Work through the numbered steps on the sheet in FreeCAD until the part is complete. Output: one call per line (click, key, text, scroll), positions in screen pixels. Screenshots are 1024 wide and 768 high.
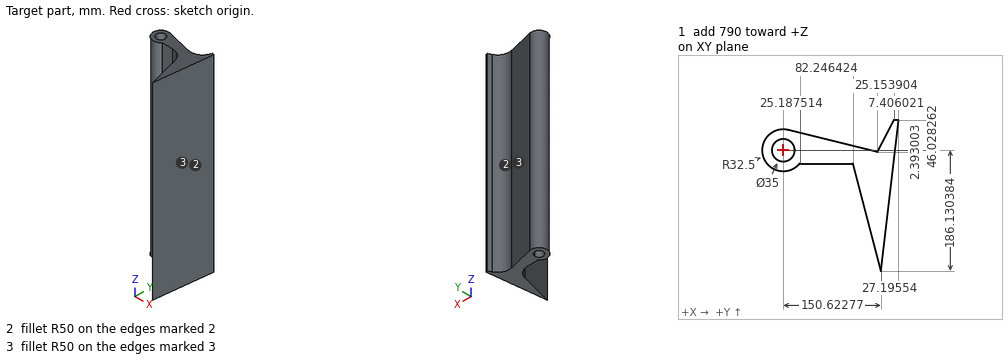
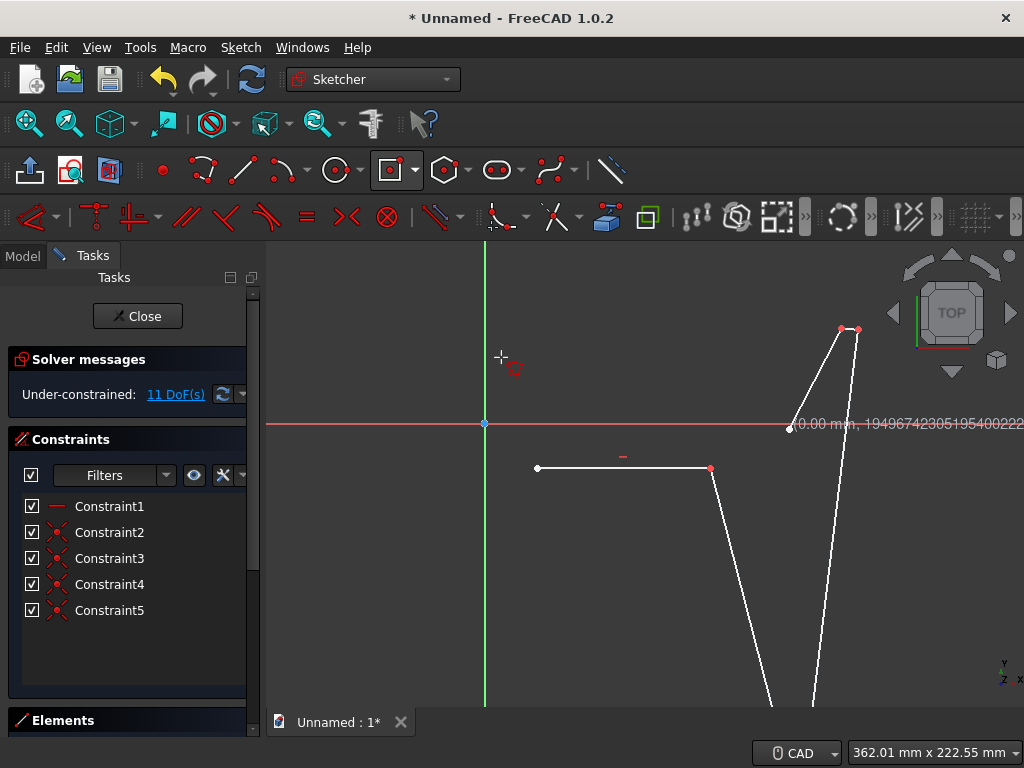
click(501, 358)
right_click(501, 358)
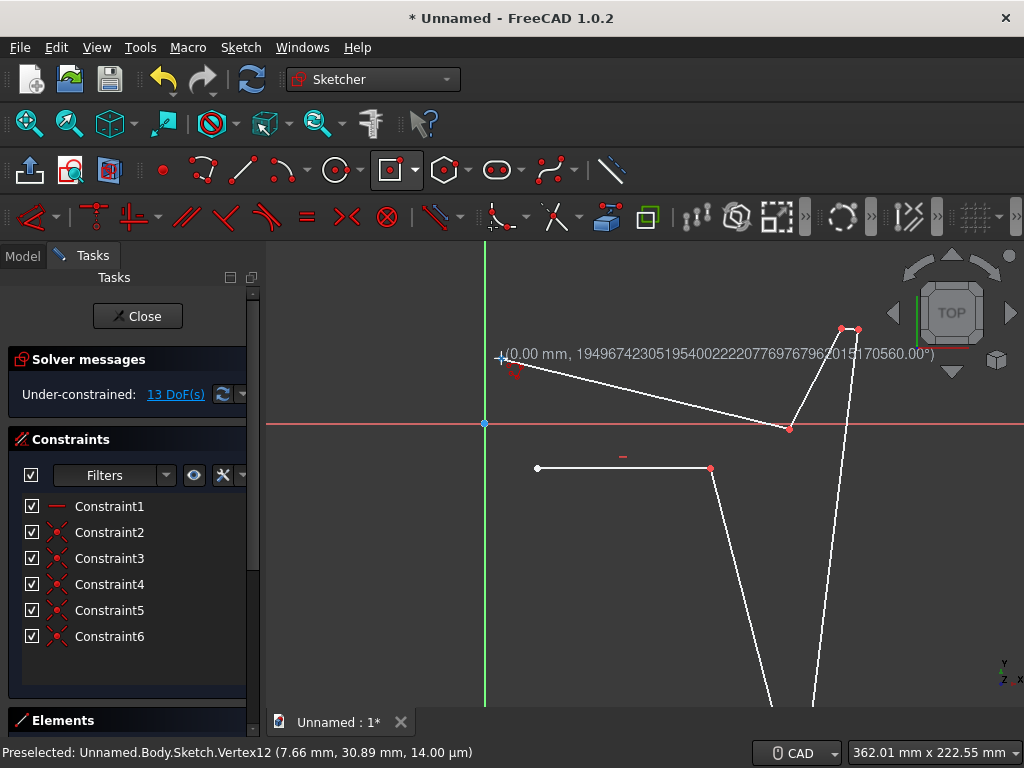
key(g)
key(3)
key(a)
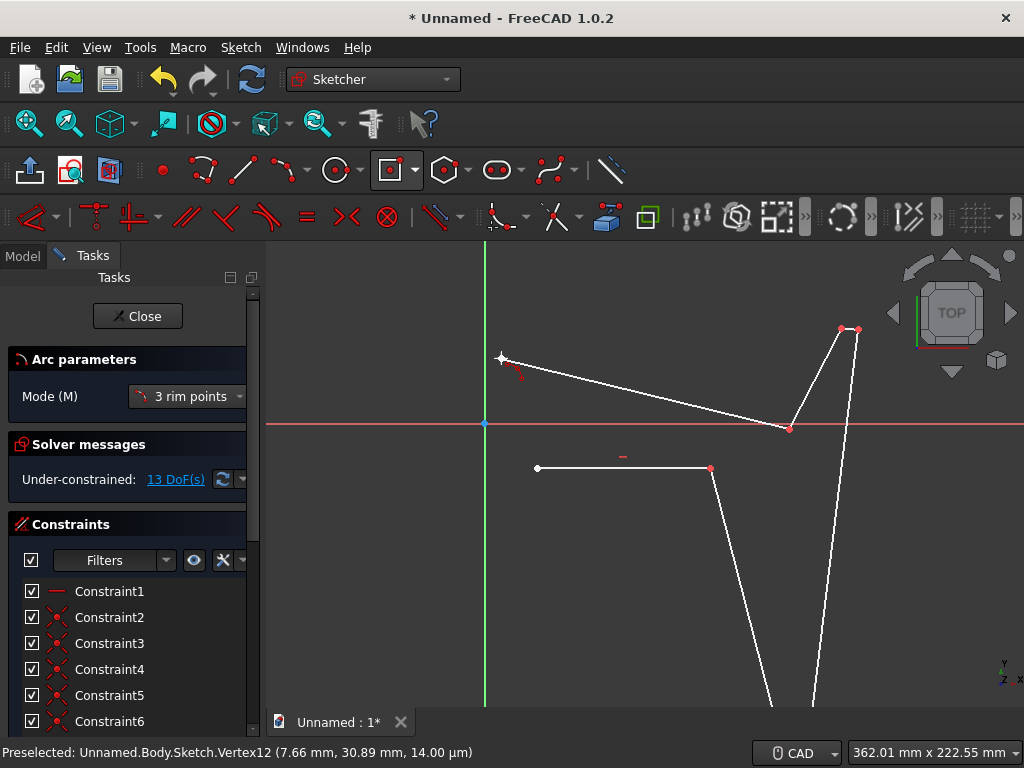
click(501, 359)
click(537, 468)
click(435, 470)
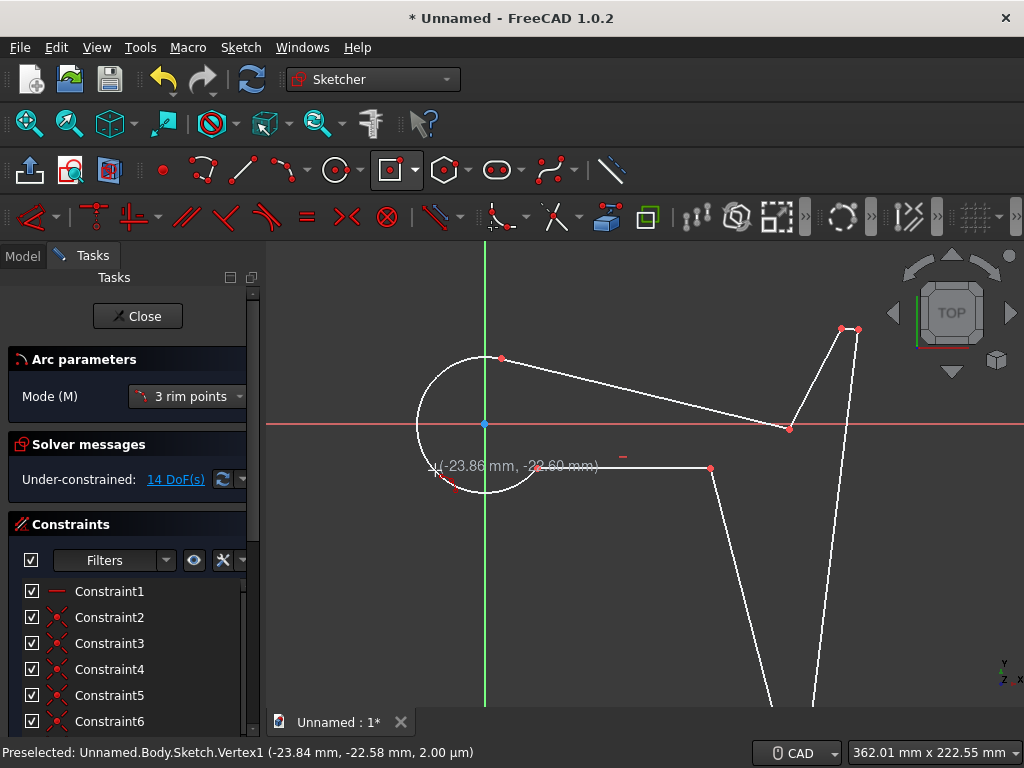
key(g)
key(c)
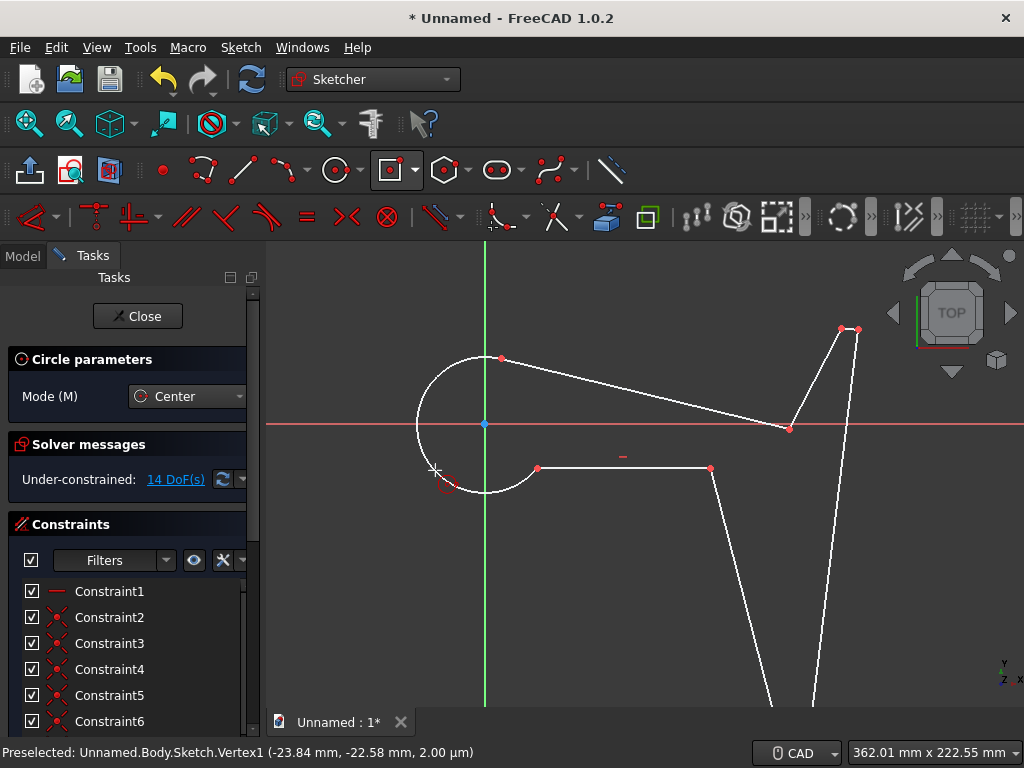
click(485, 424)
move(511, 398)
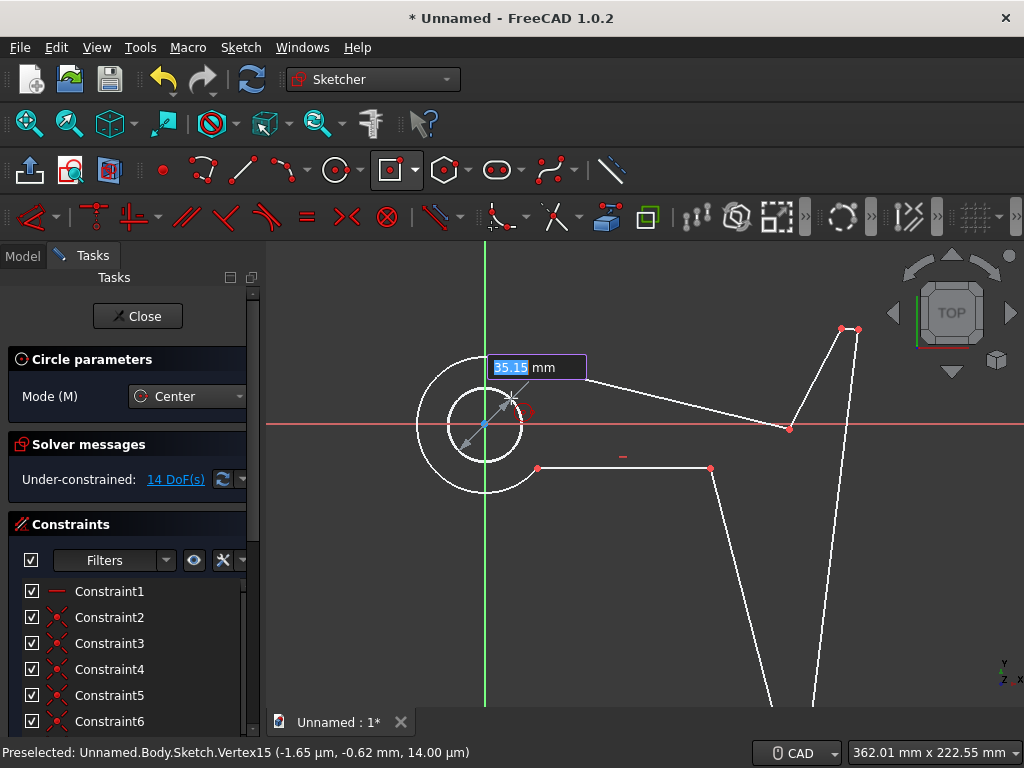
text(35)
key(Return)
key(Escape)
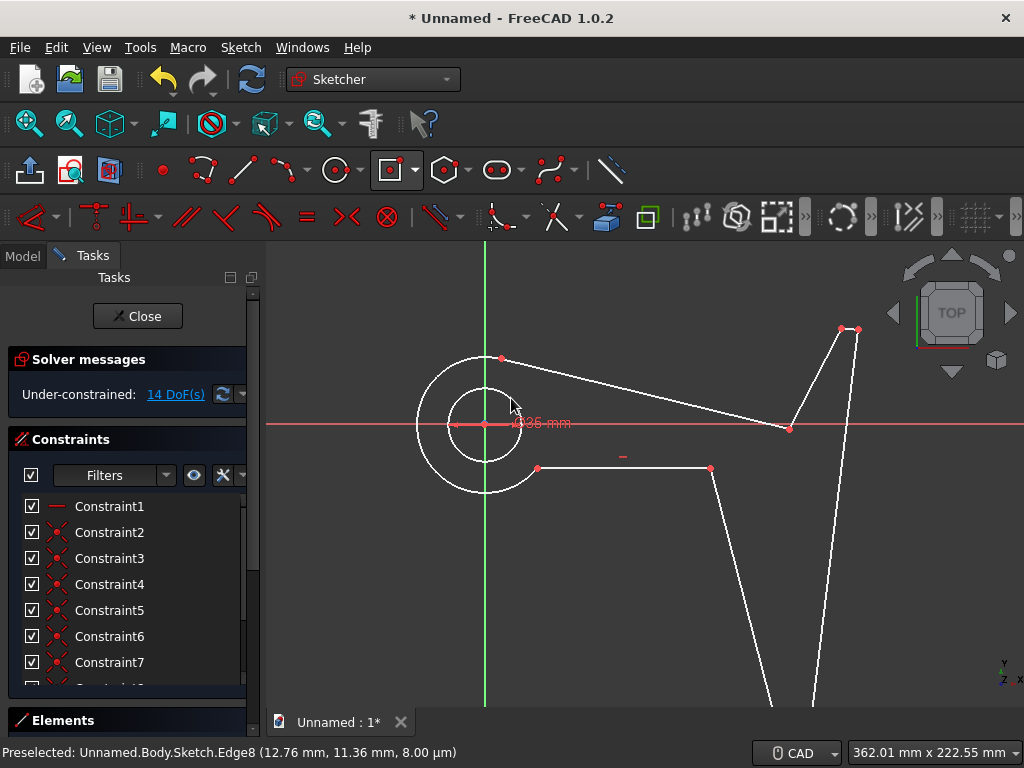
click(703, 408)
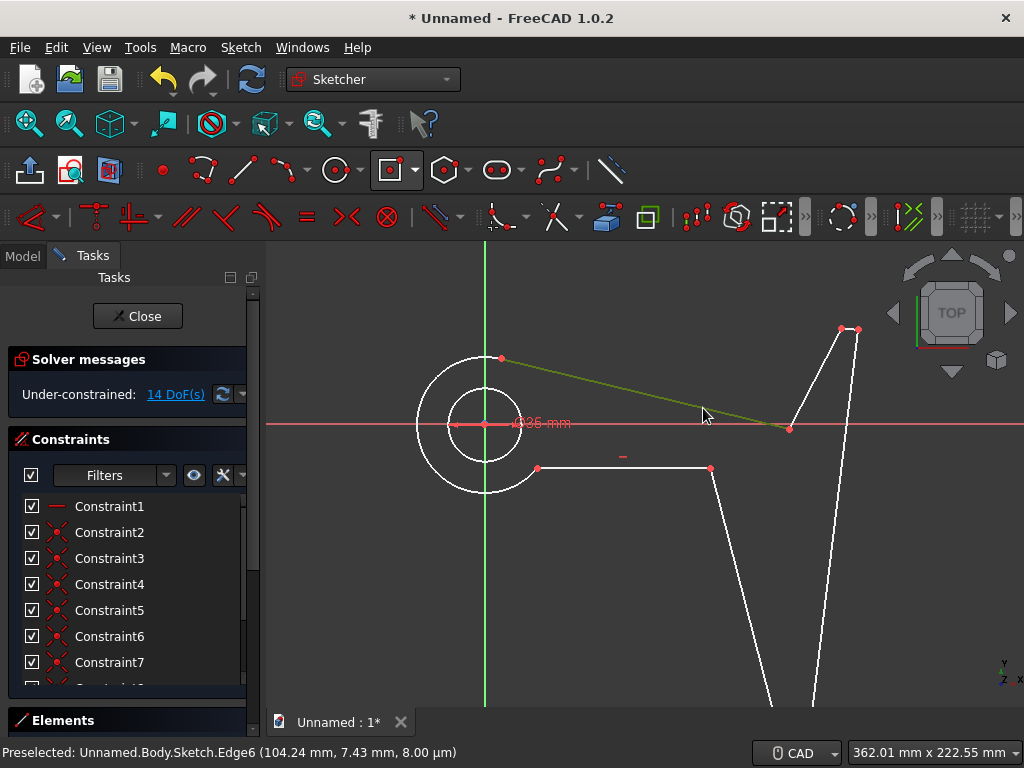
click(426, 391)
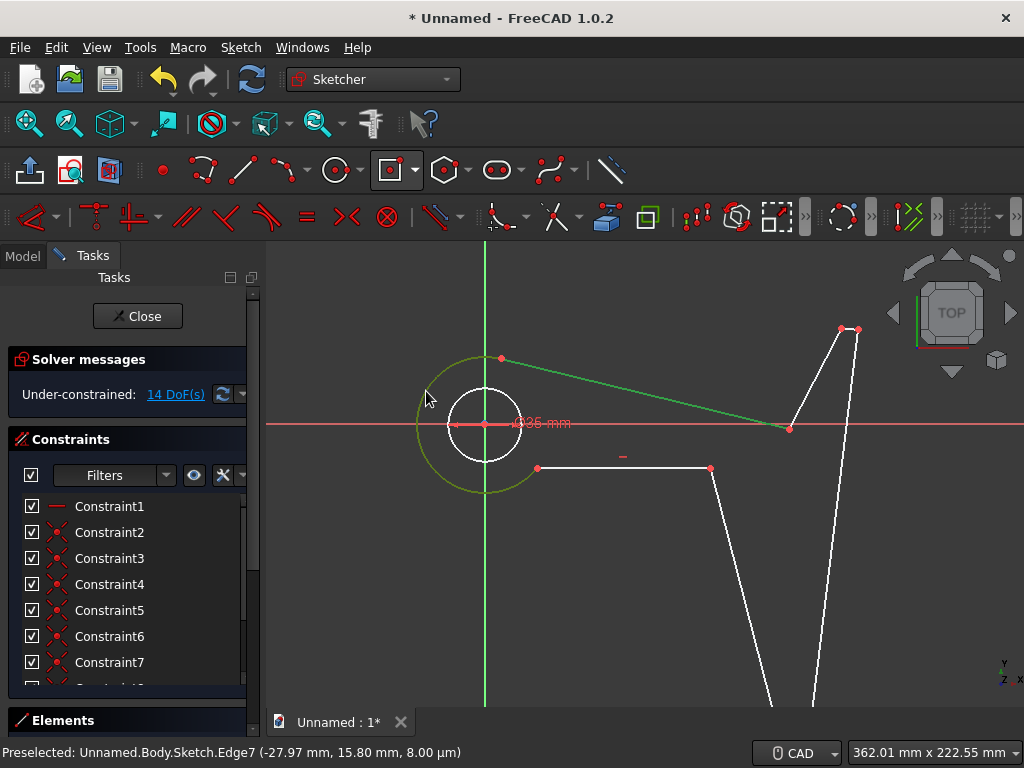
key(t)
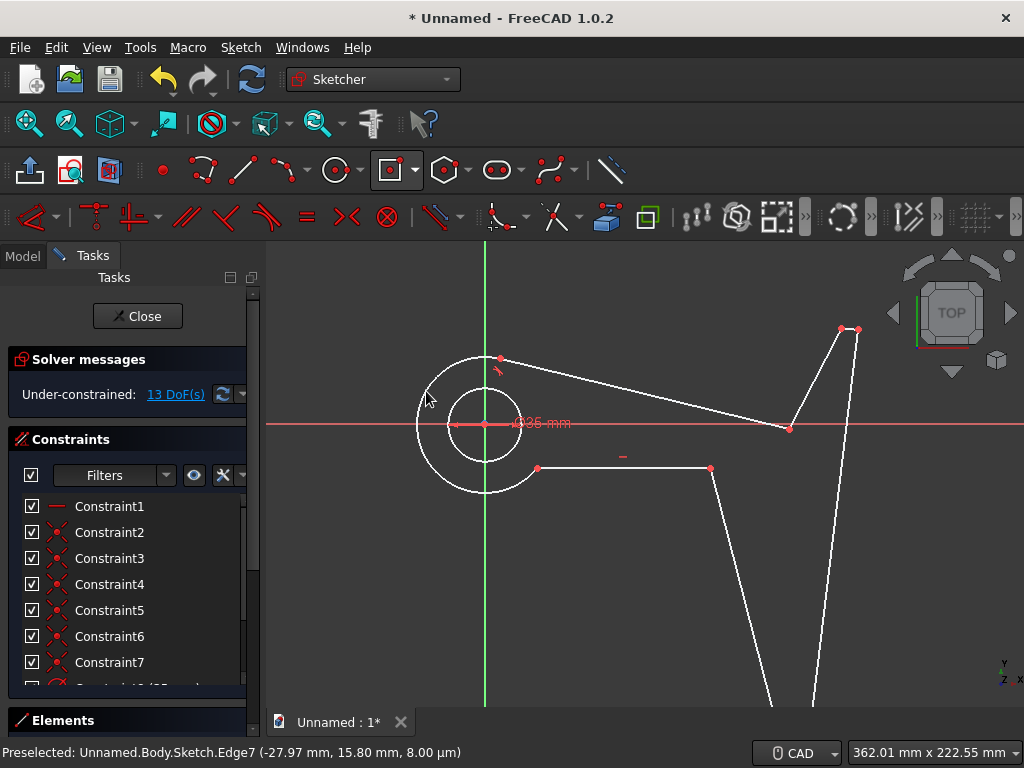
scroll(850, 329, up, 3)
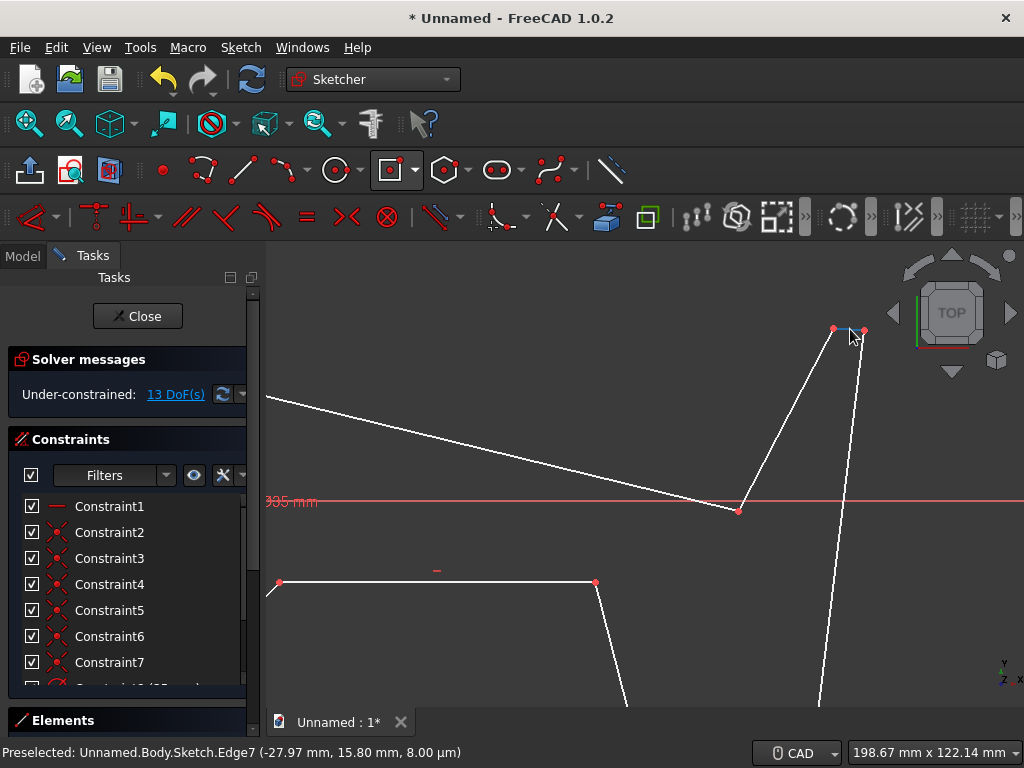
click(849, 329)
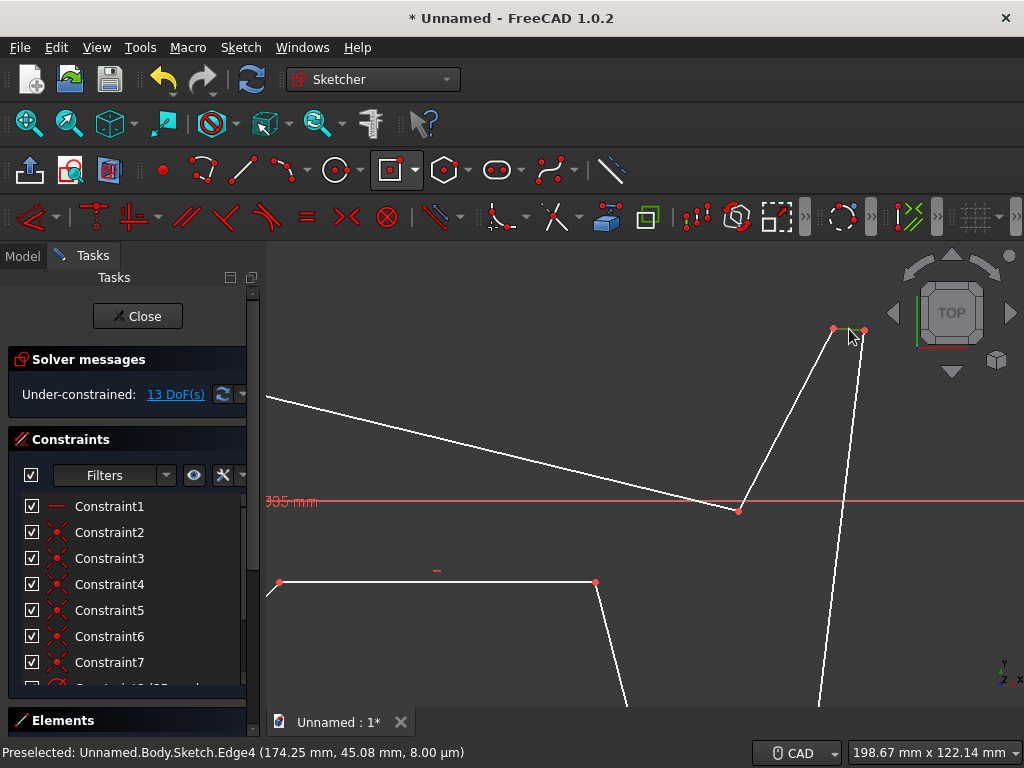
key(h)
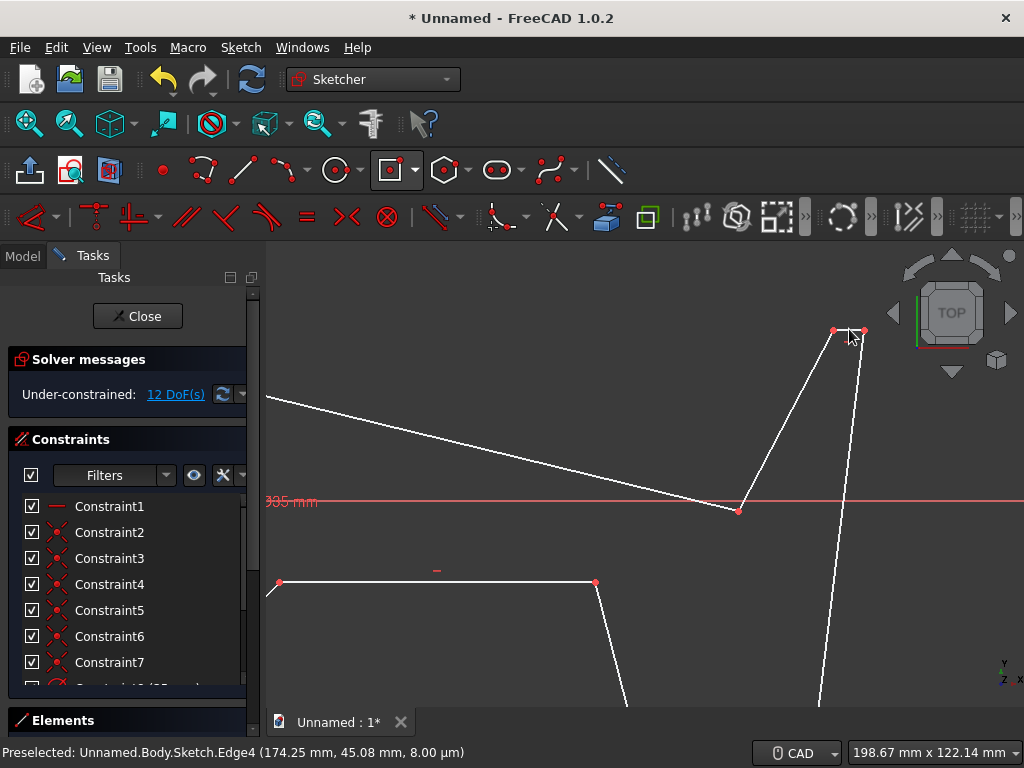
scroll(625, 347, down, 6)